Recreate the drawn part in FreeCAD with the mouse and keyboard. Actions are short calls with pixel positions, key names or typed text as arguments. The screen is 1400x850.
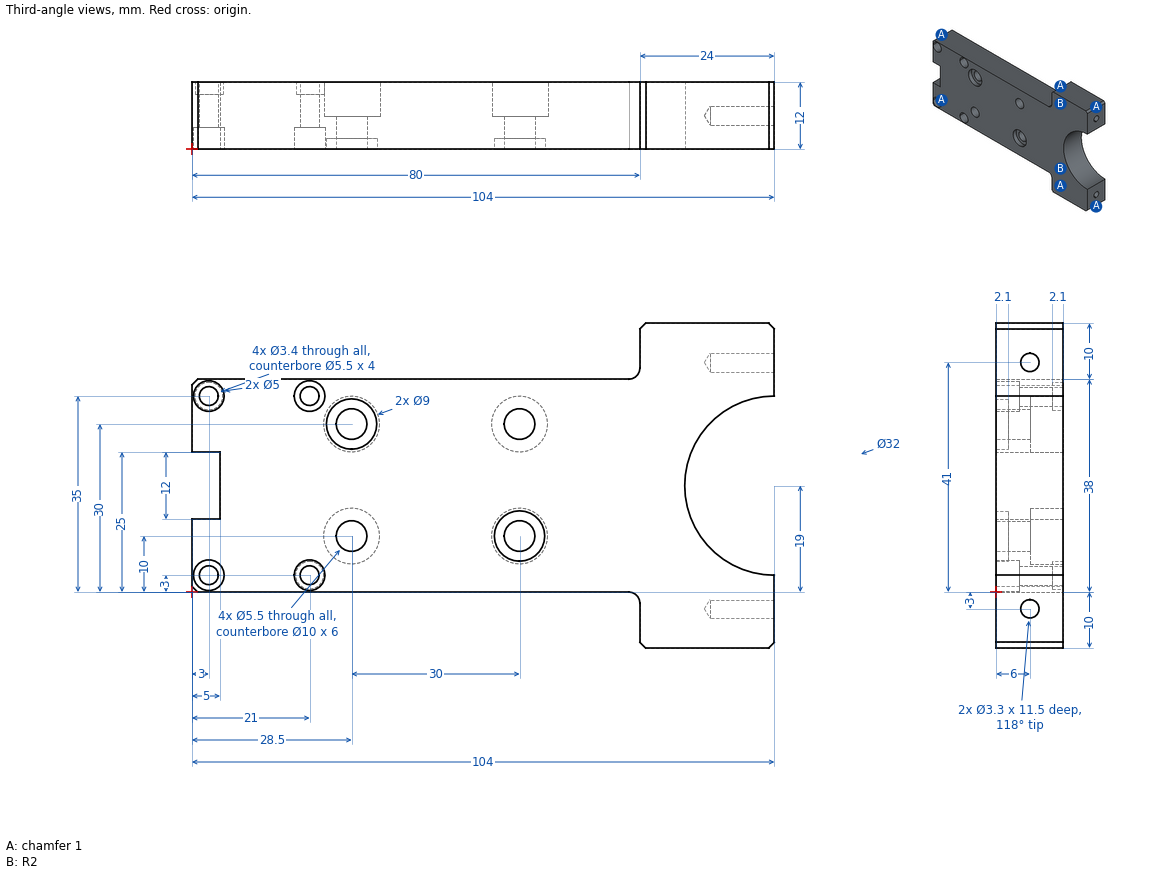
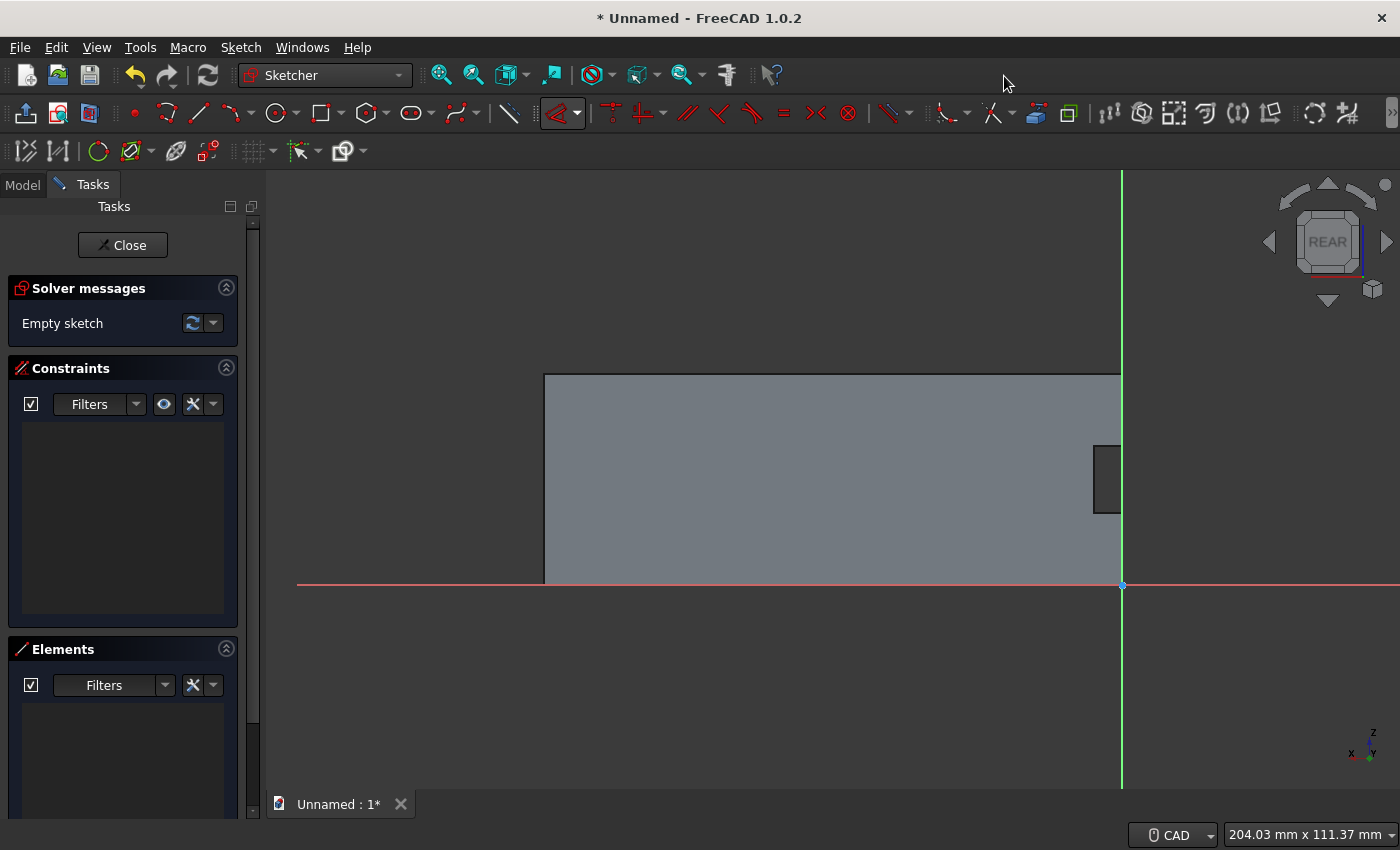
scroll(364, 480, up, 4)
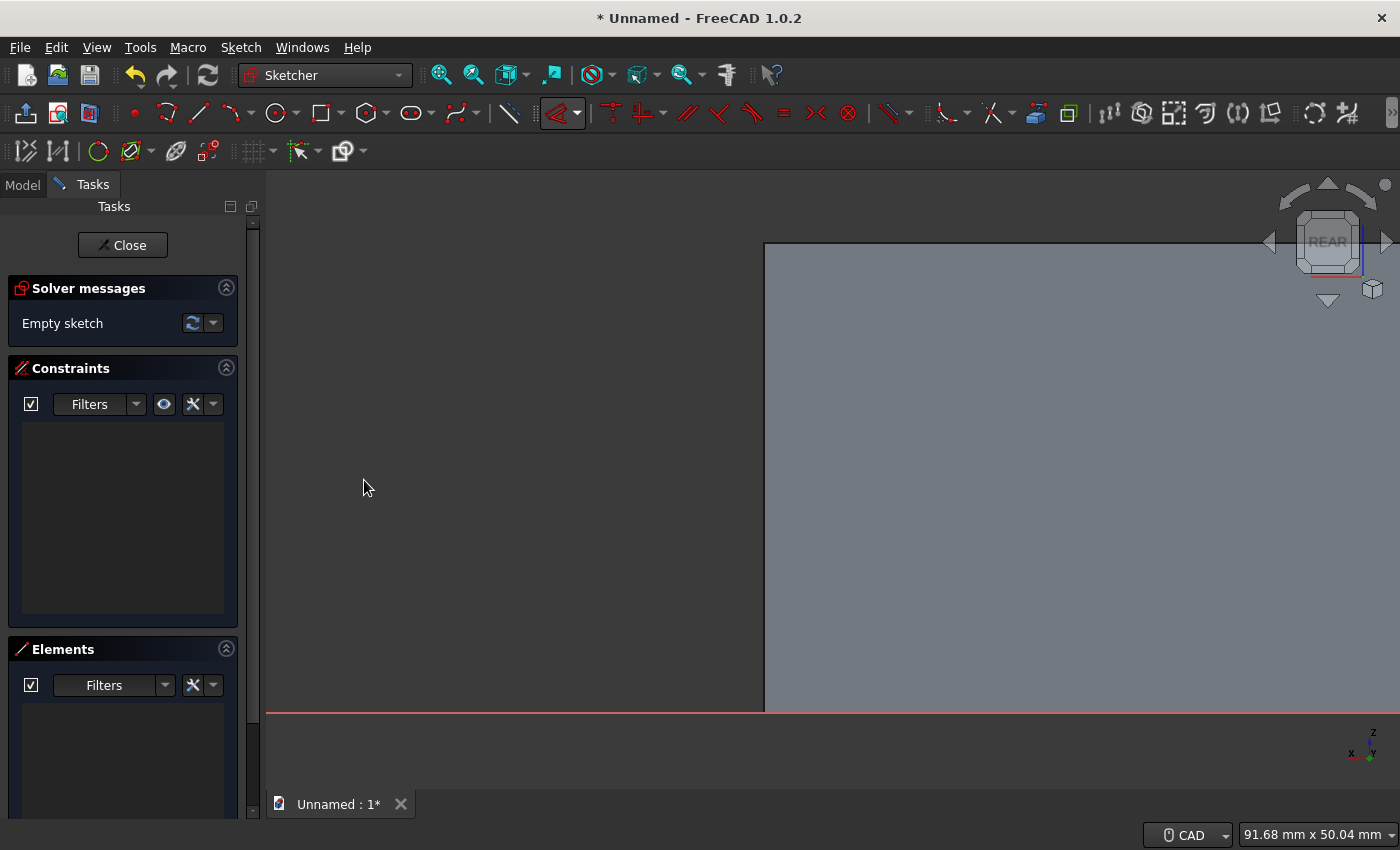
click(276, 114)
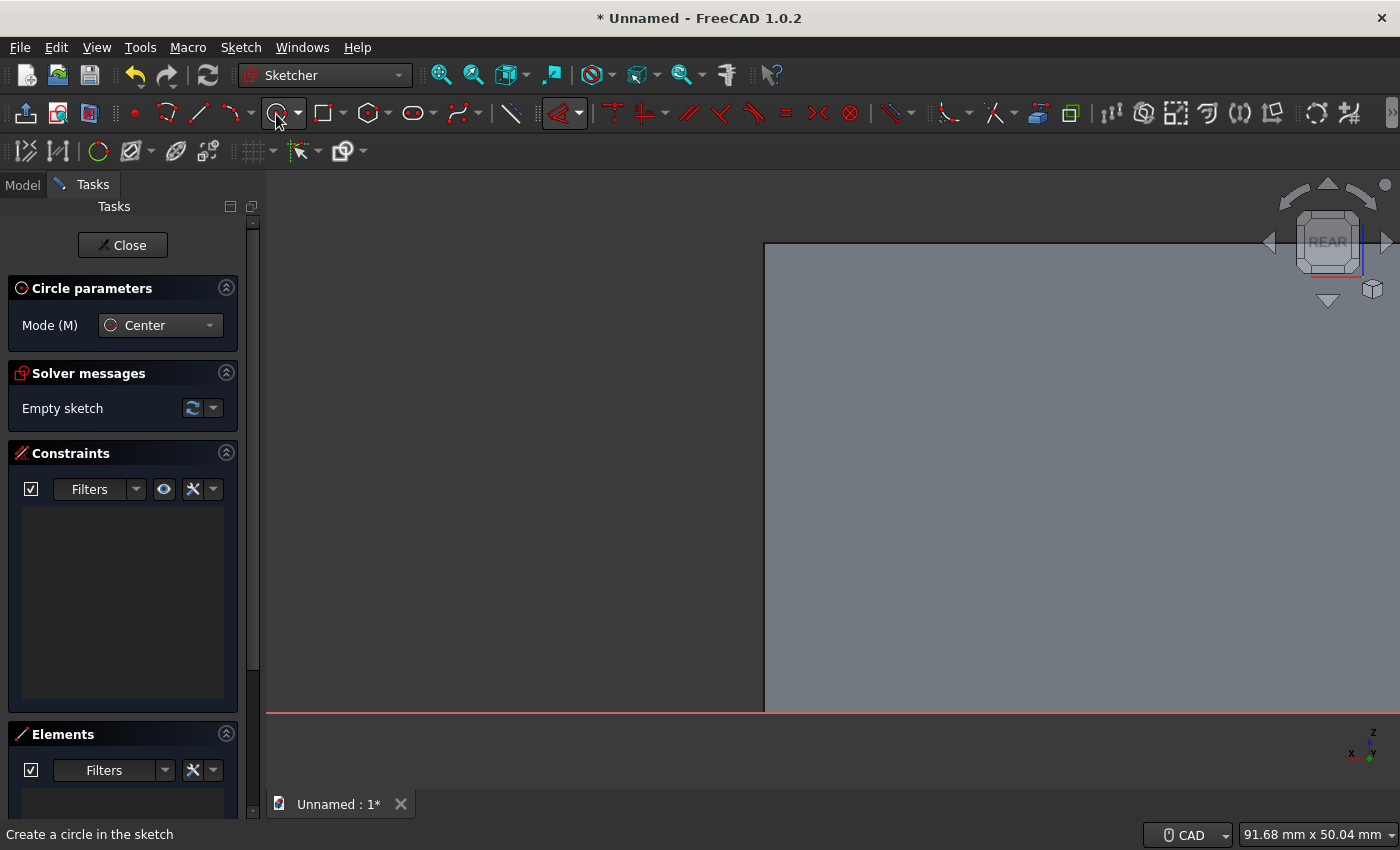
click(764, 478)
click(904, 338)
key(Escape)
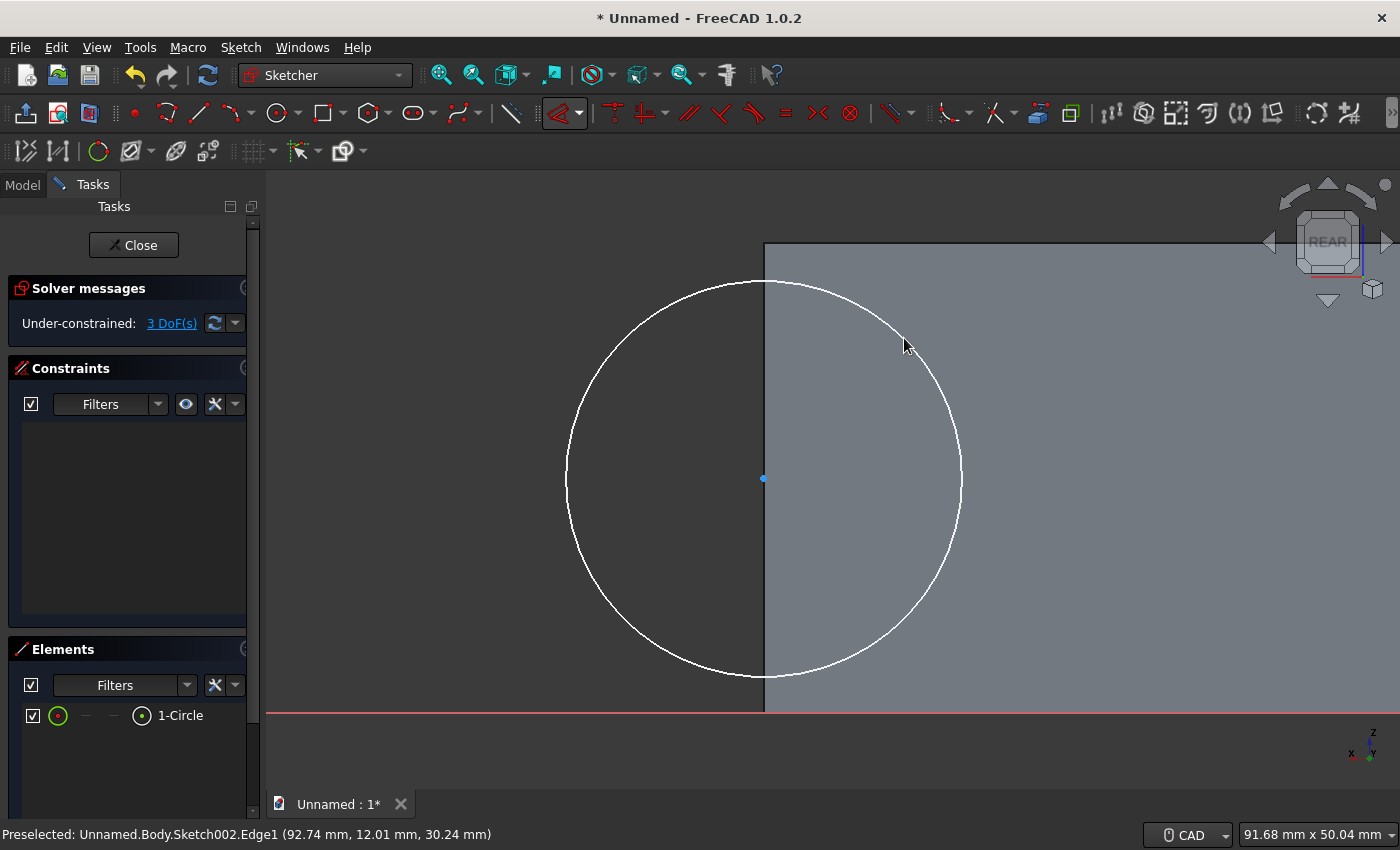
click(904, 339)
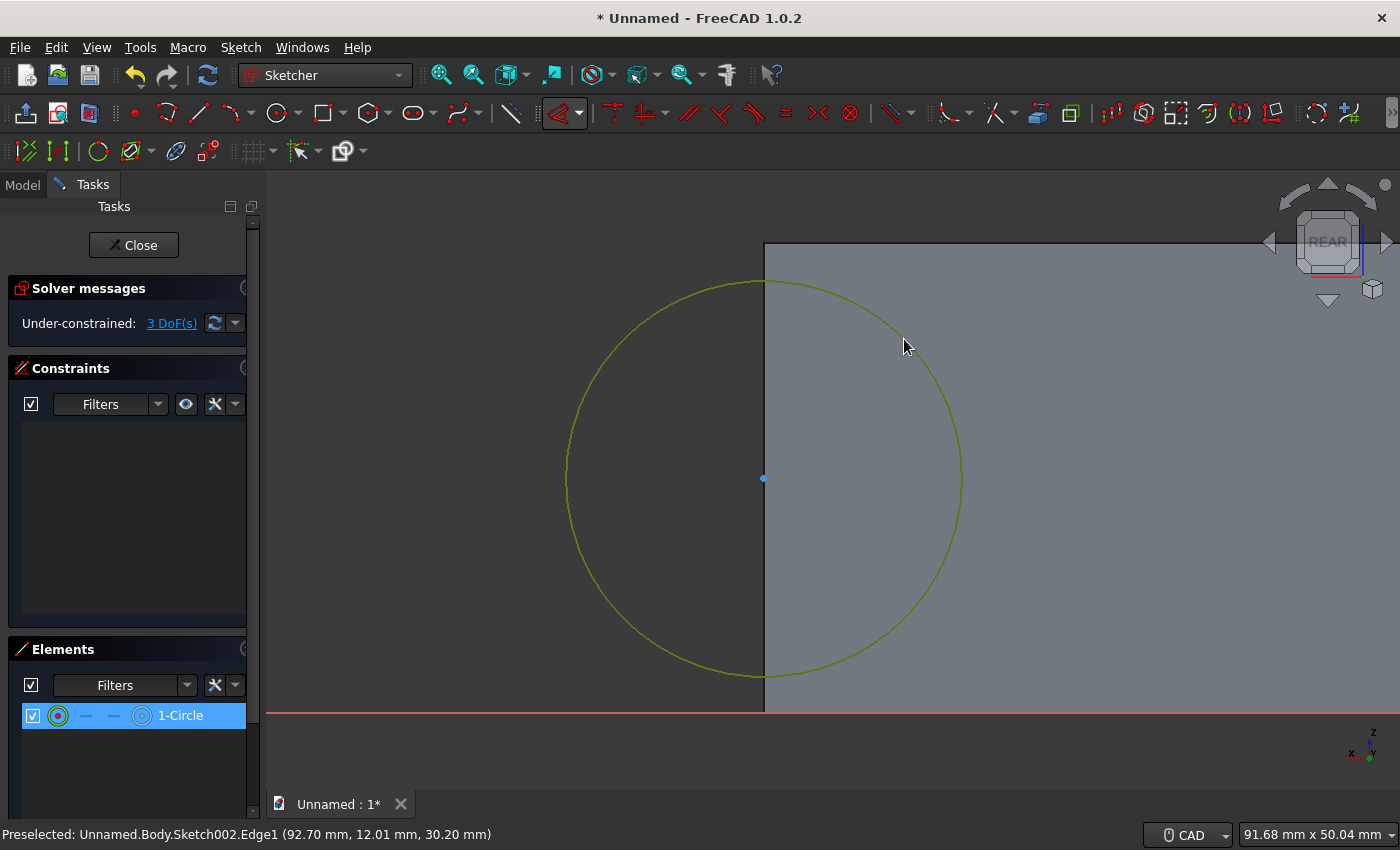
click(582, 114)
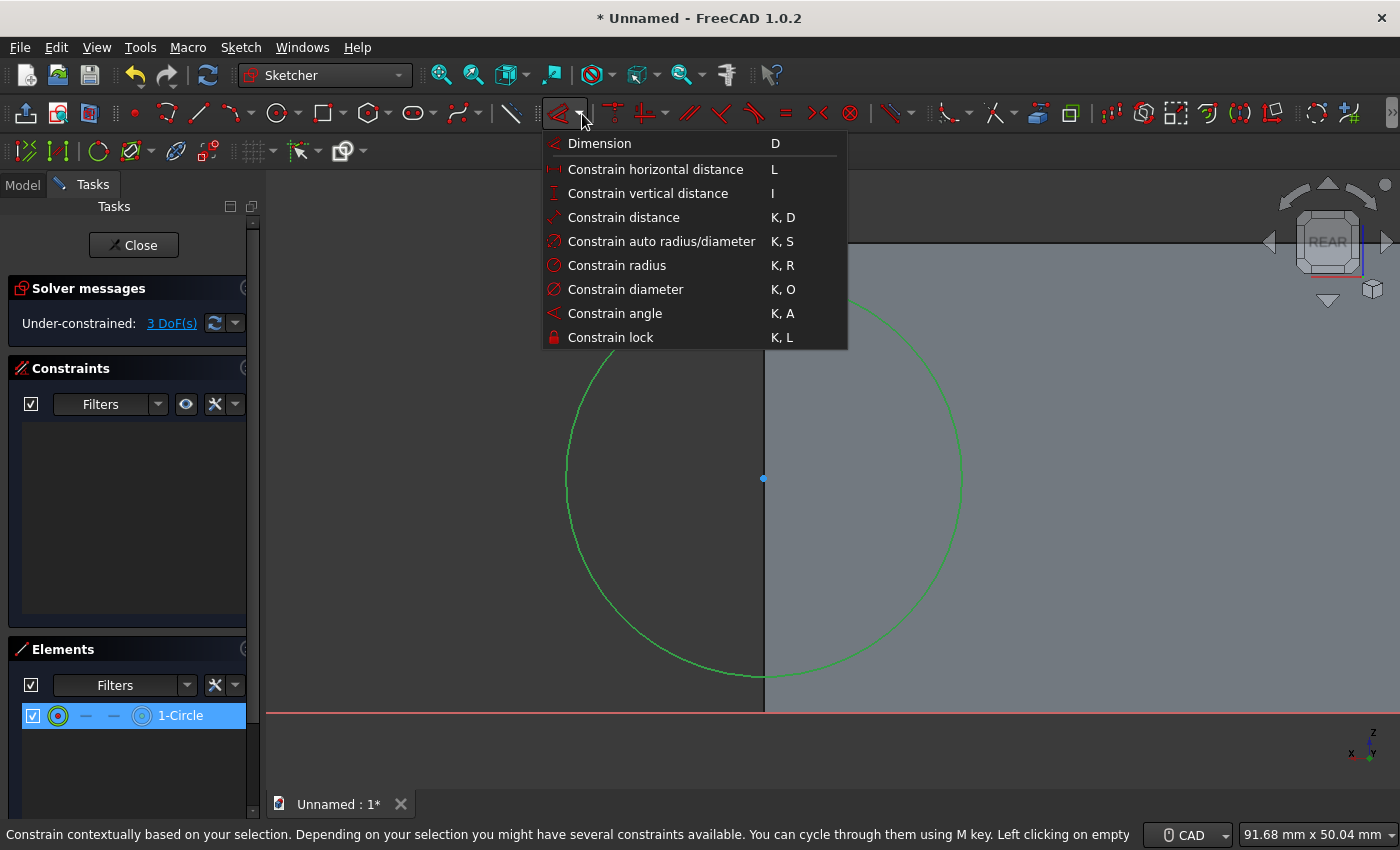
click(695, 289)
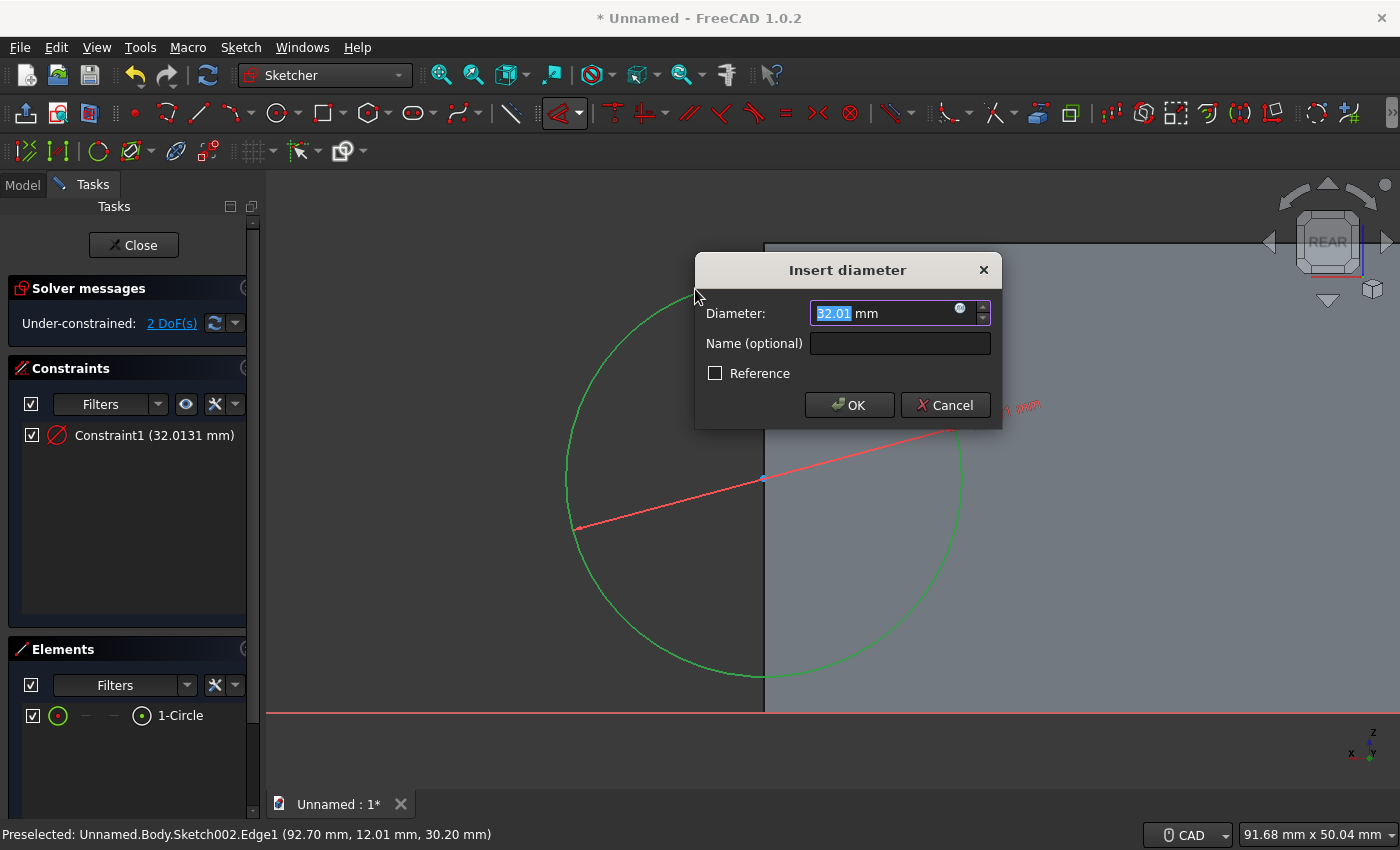
text(32)
key(Return)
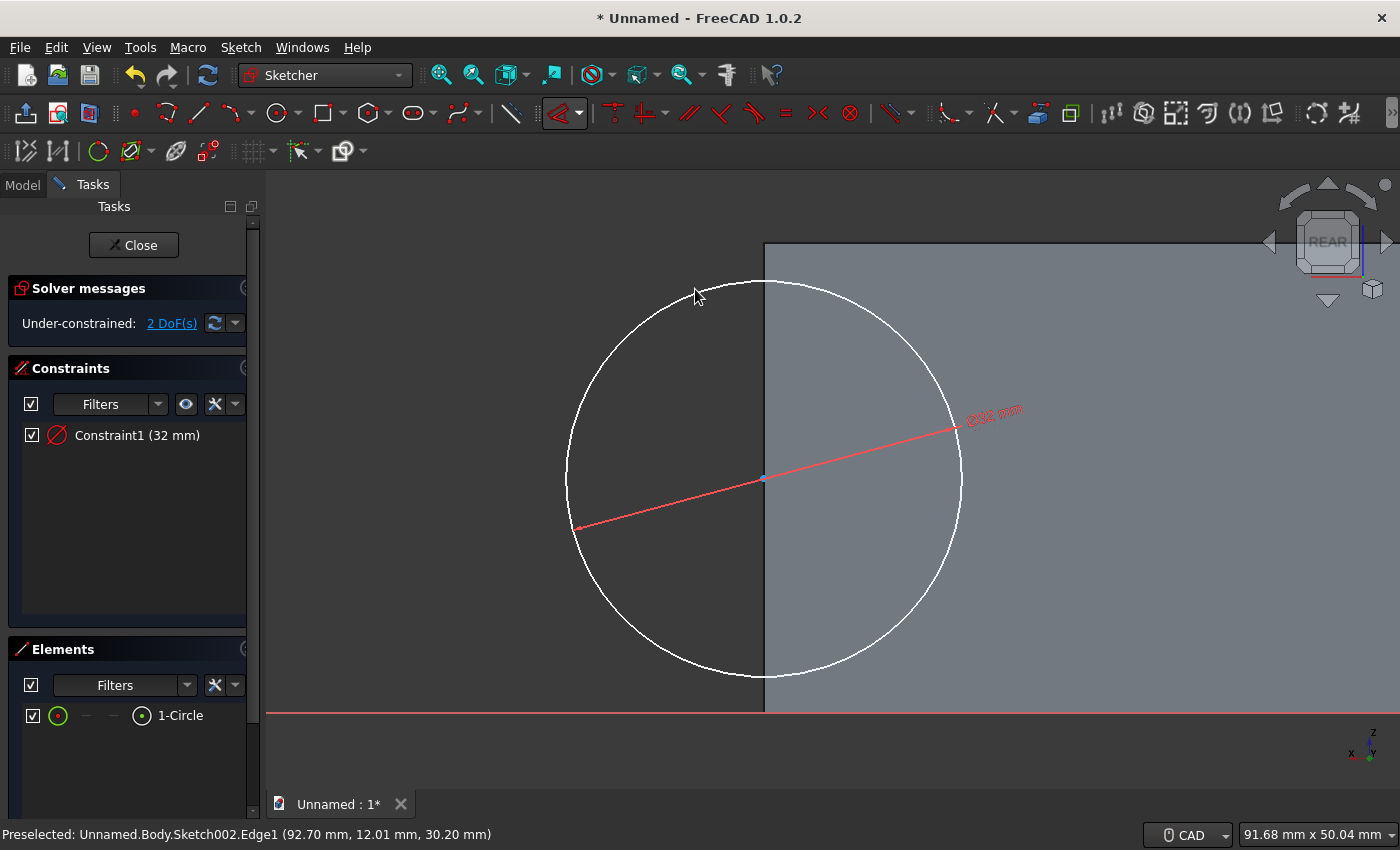
click(764, 479)